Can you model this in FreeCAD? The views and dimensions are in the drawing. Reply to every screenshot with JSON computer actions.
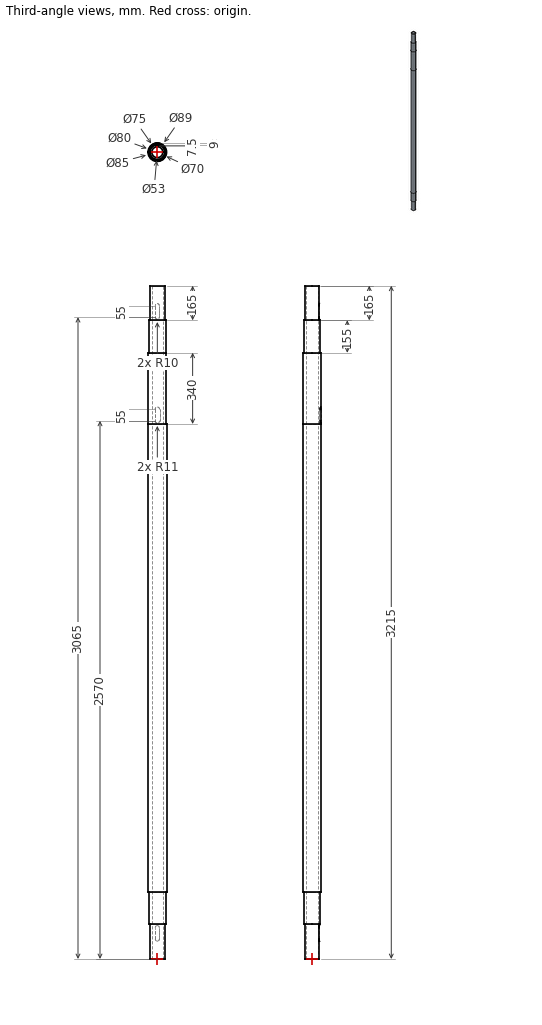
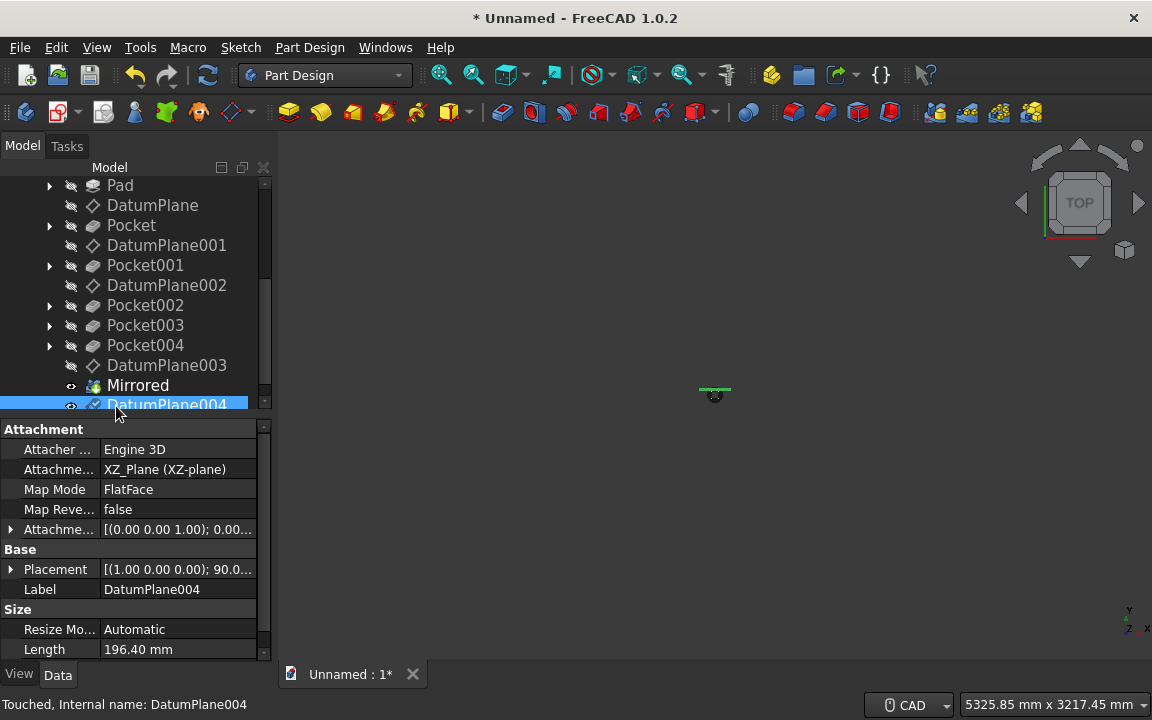
{"action": "left_click", "coordinate": [58, 112]}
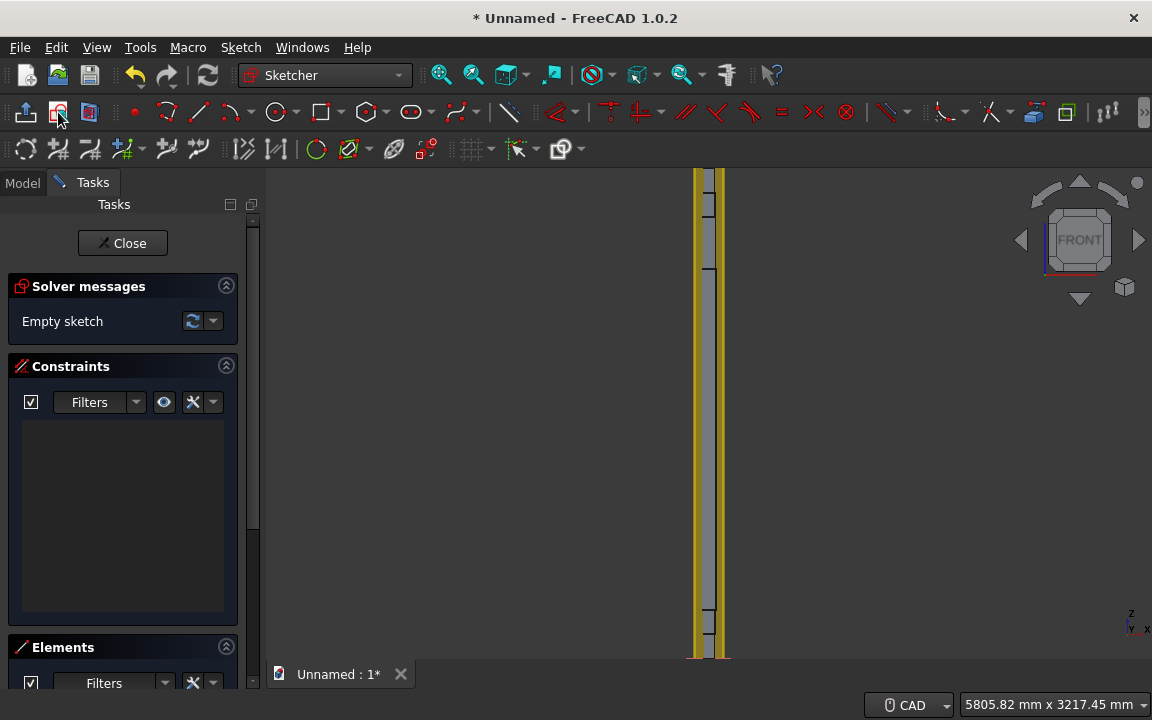
{"action": "left_click", "coordinate": [90, 112]}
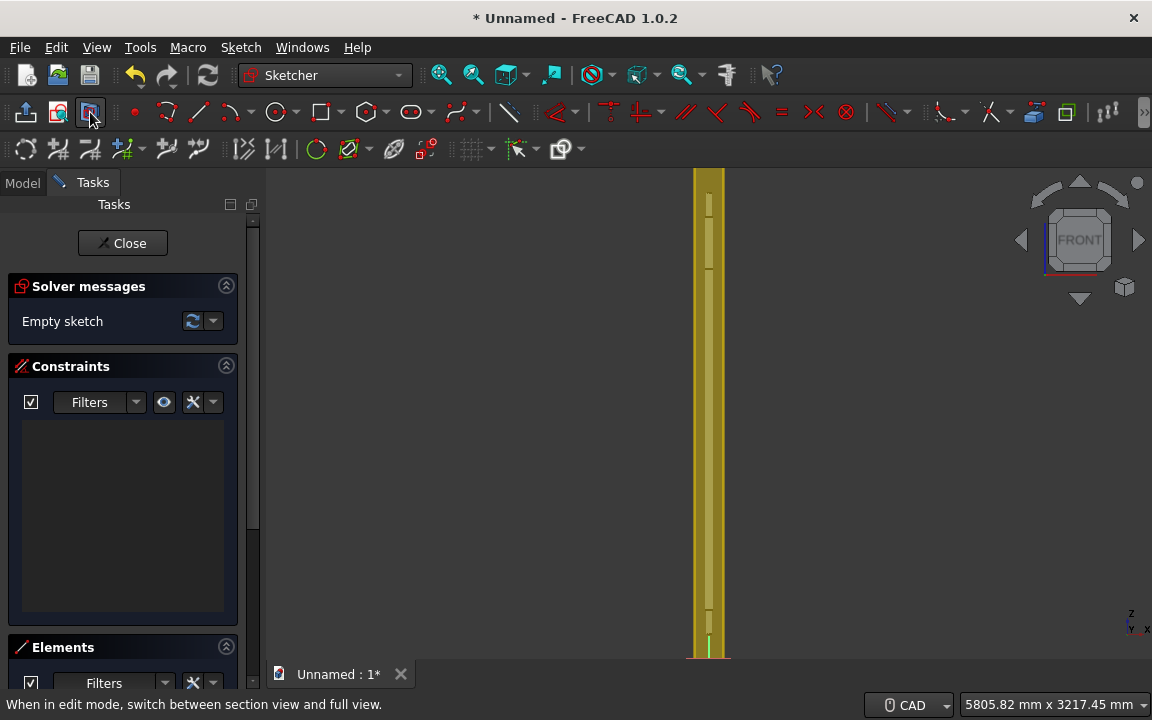
{"action": "scroll", "coordinate": [640, 414], "scroll_direction": "down", "scroll_amount": 5}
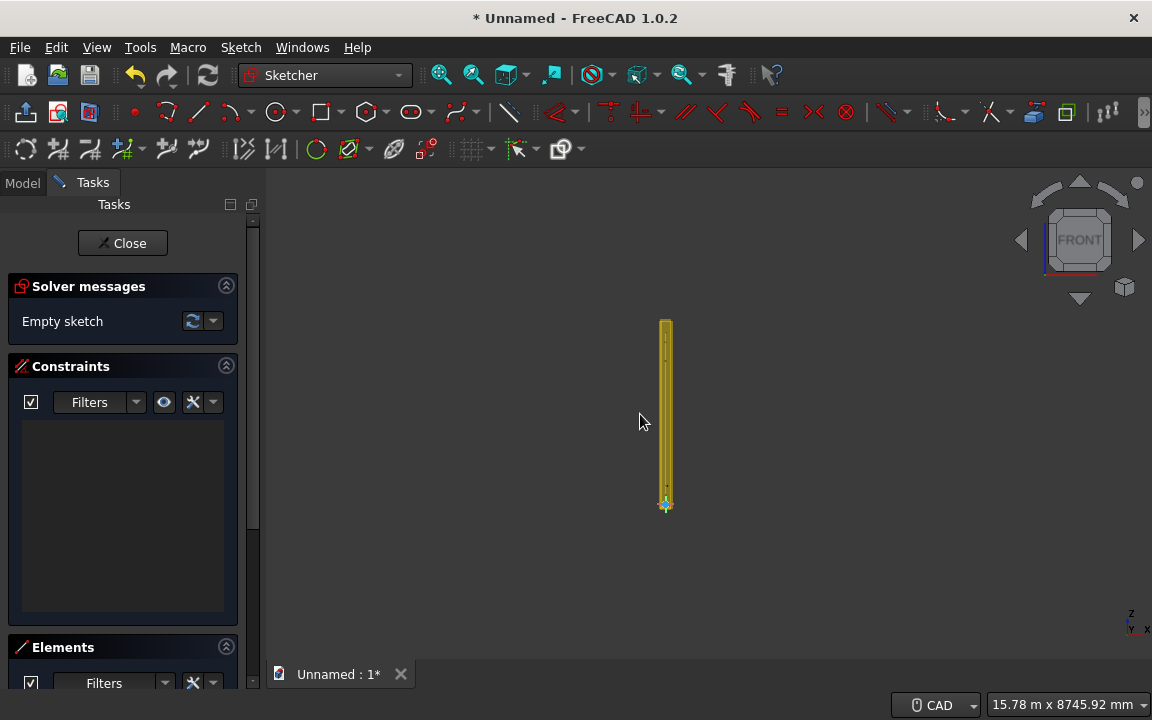
{"action": "scroll", "coordinate": [667, 326], "scroll_direction": "up", "scroll_amount": 15}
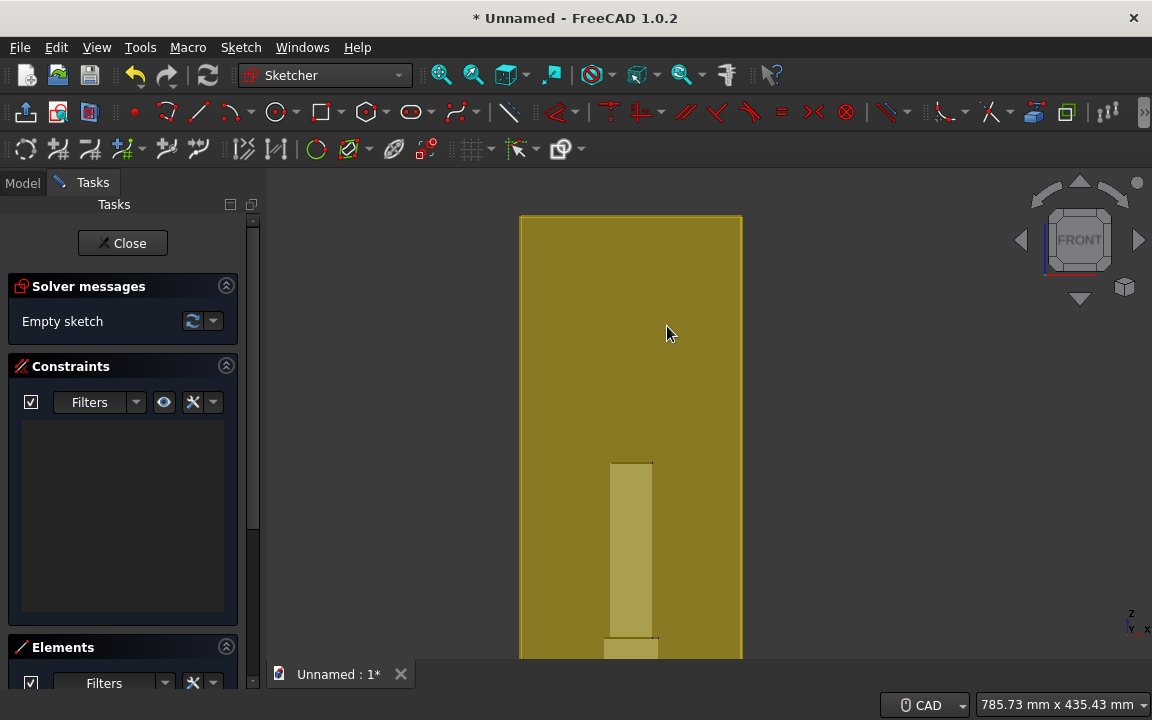
{"action": "scroll", "coordinate": [627, 416], "scroll_direction": "up", "scroll_amount": 6}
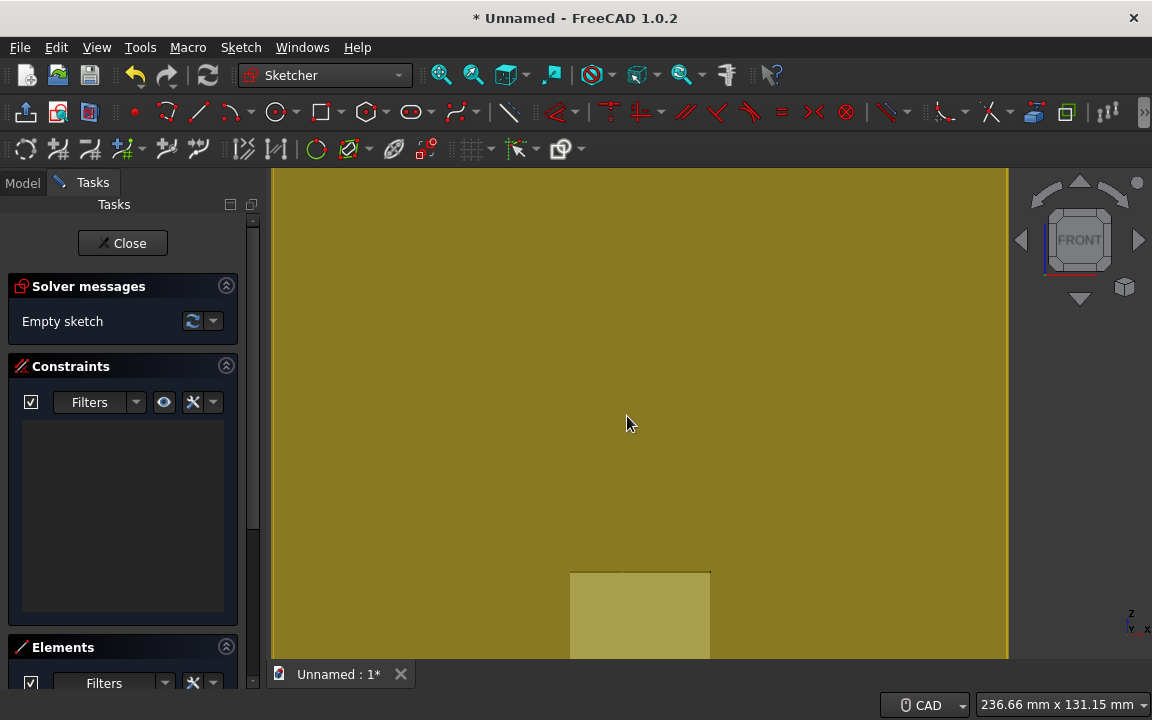
{"action": "left_click", "coordinate": [412, 112]}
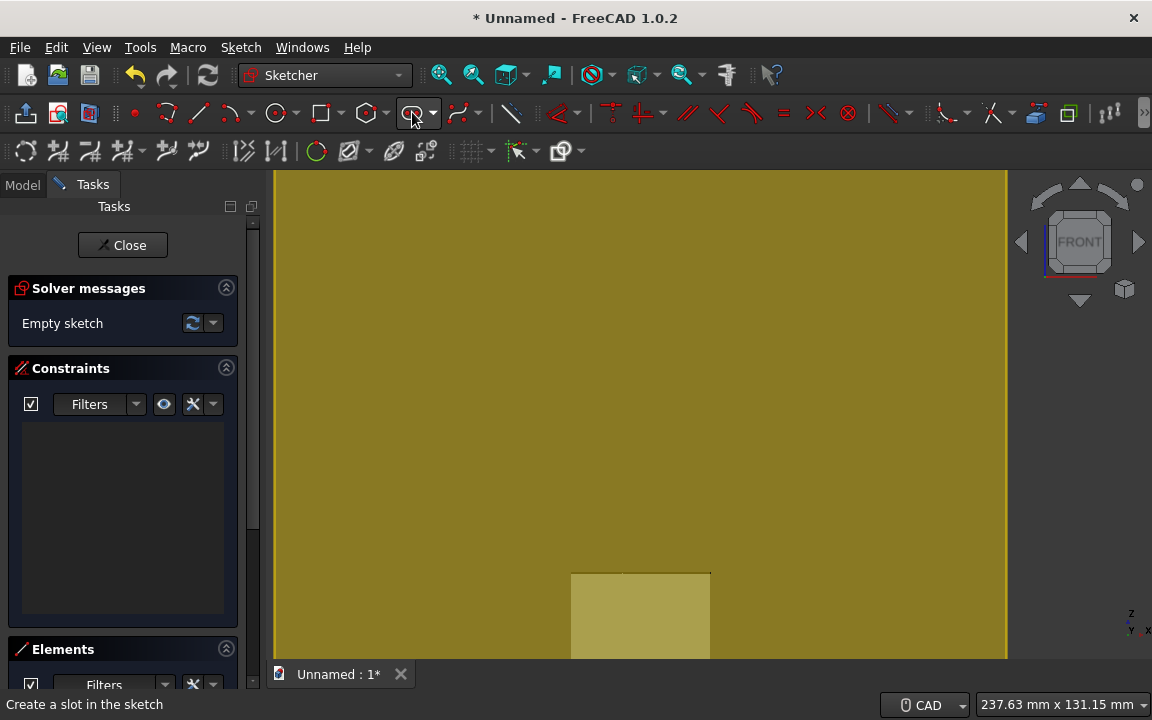
{"action": "left_click", "coordinate": [640, 517]}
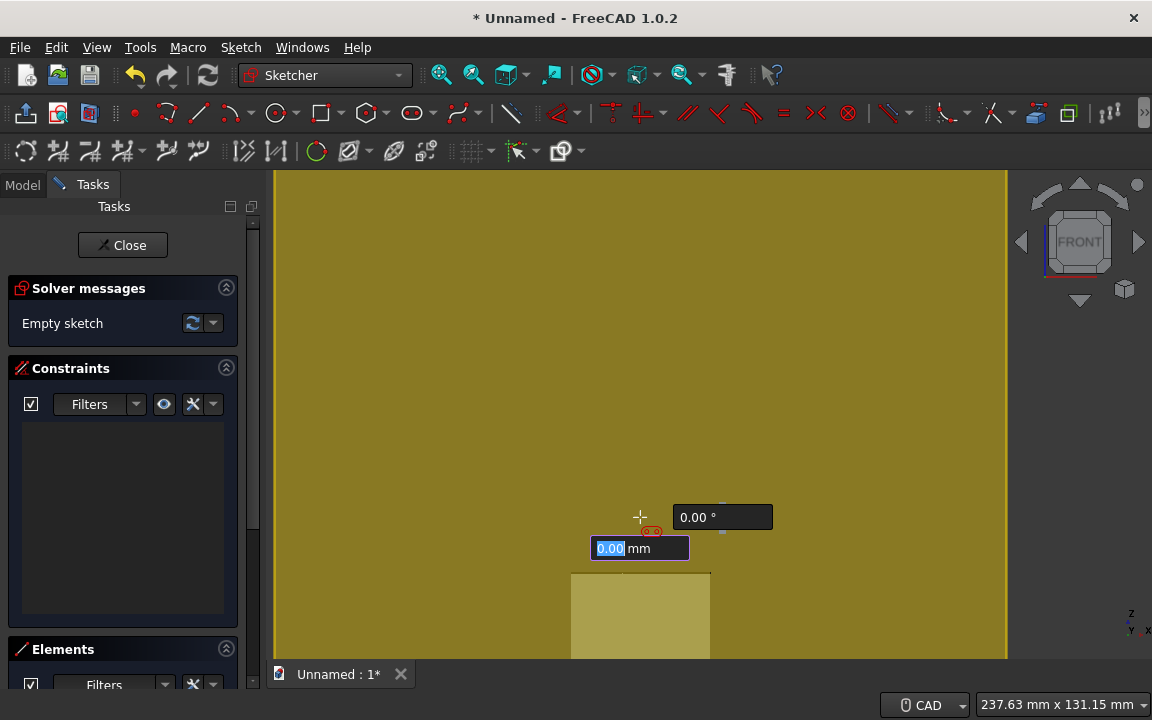
{"action": "left_click", "coordinate": [649, 312]}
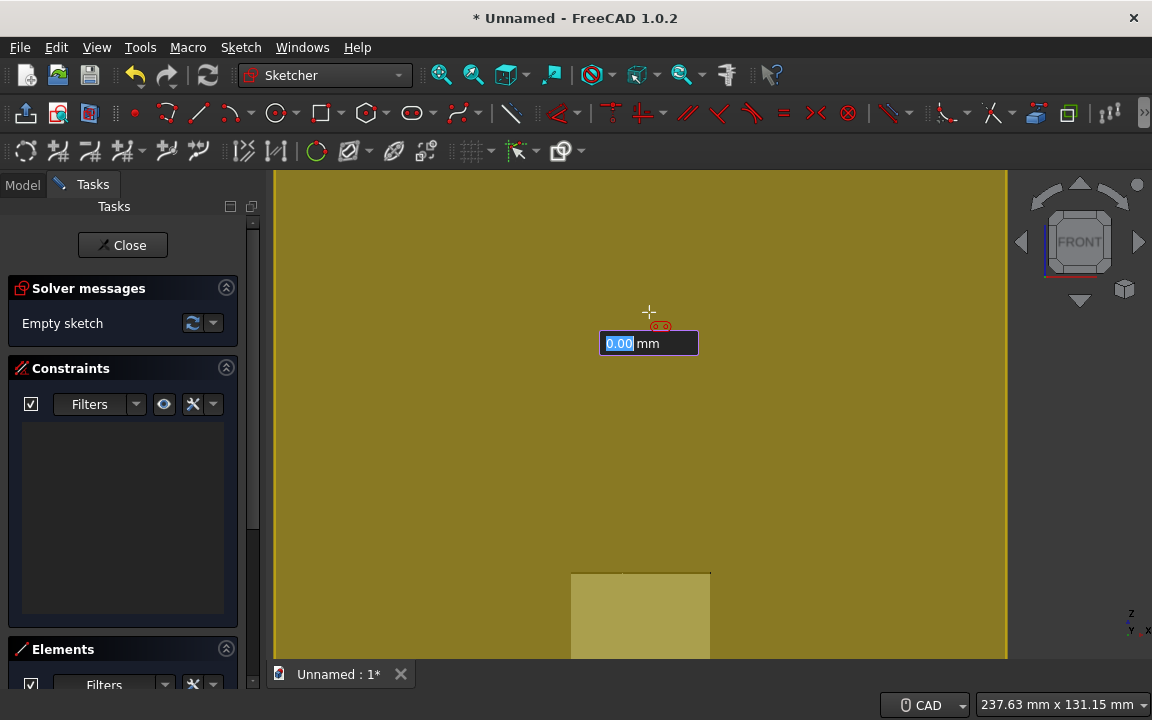
{"action": "left_click", "coordinate": [678, 414]}
{"action": "key", "text": "Escape"}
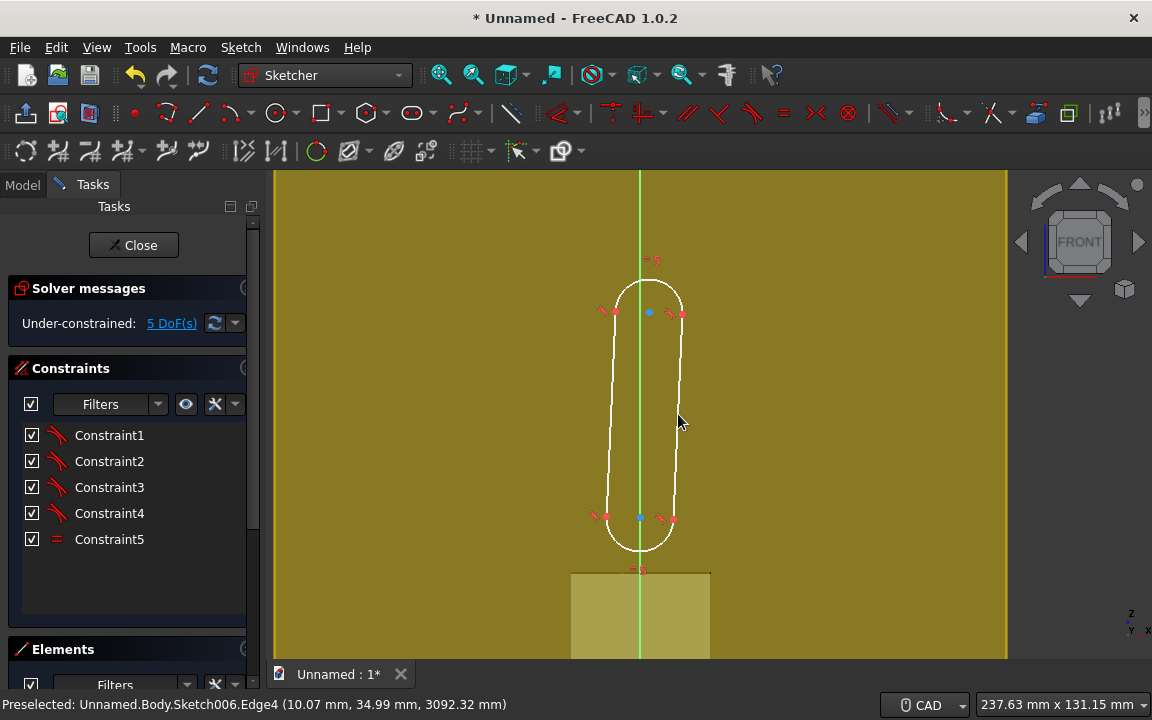
{"action": "left_click", "coordinate": [609, 455]}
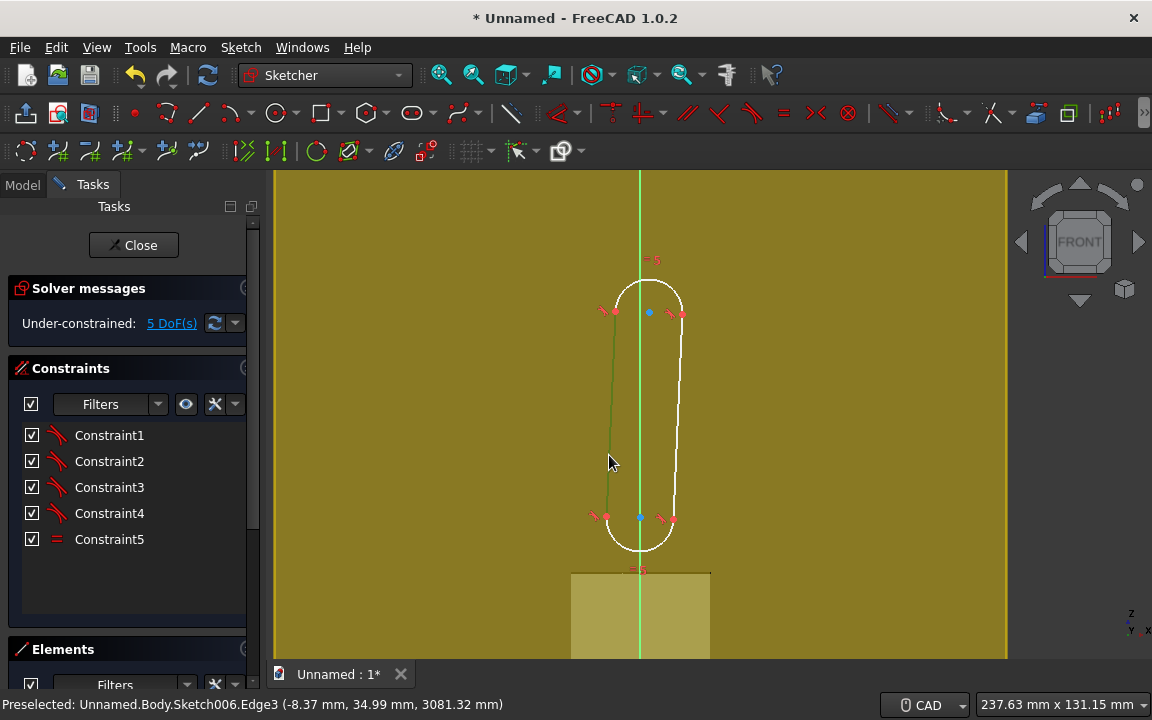
{"action": "left_click", "coordinate": [666, 114]}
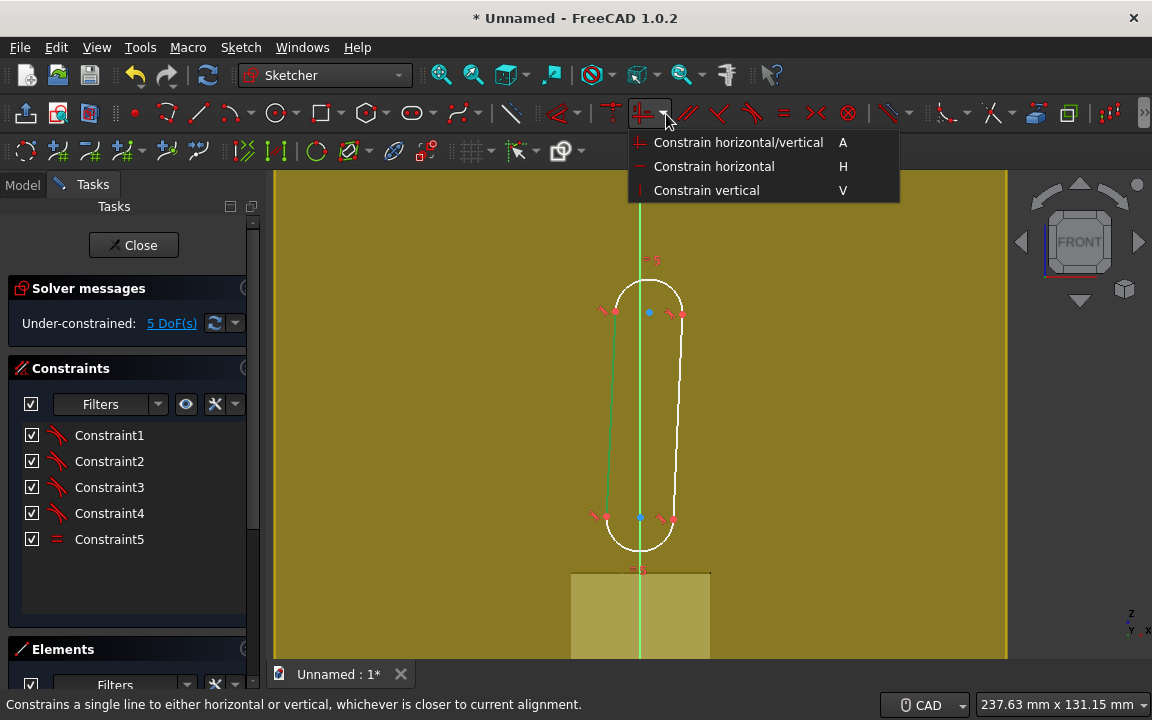
{"action": "left_click", "coordinate": [764, 190]}